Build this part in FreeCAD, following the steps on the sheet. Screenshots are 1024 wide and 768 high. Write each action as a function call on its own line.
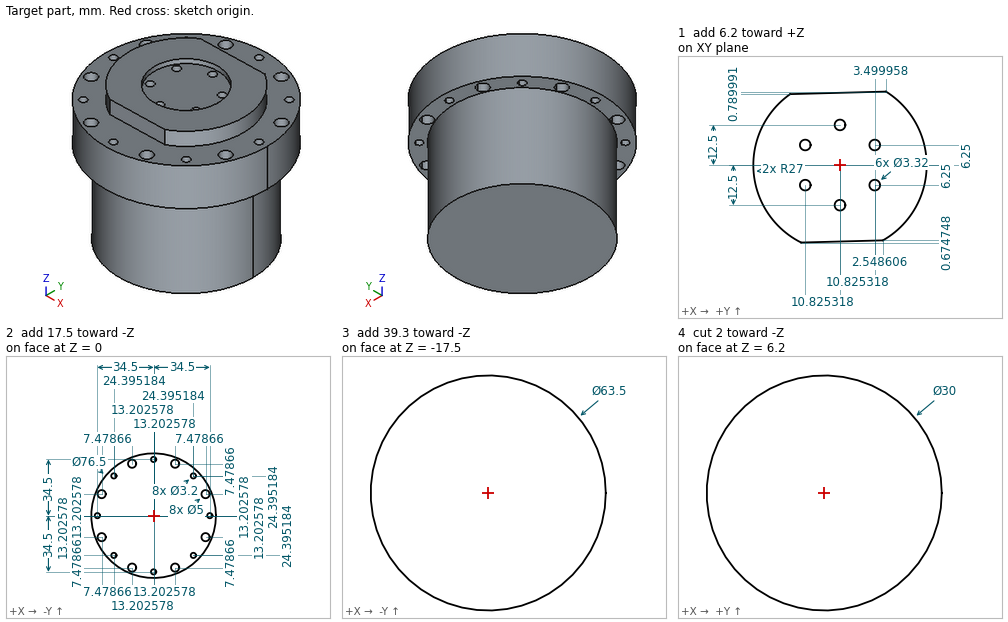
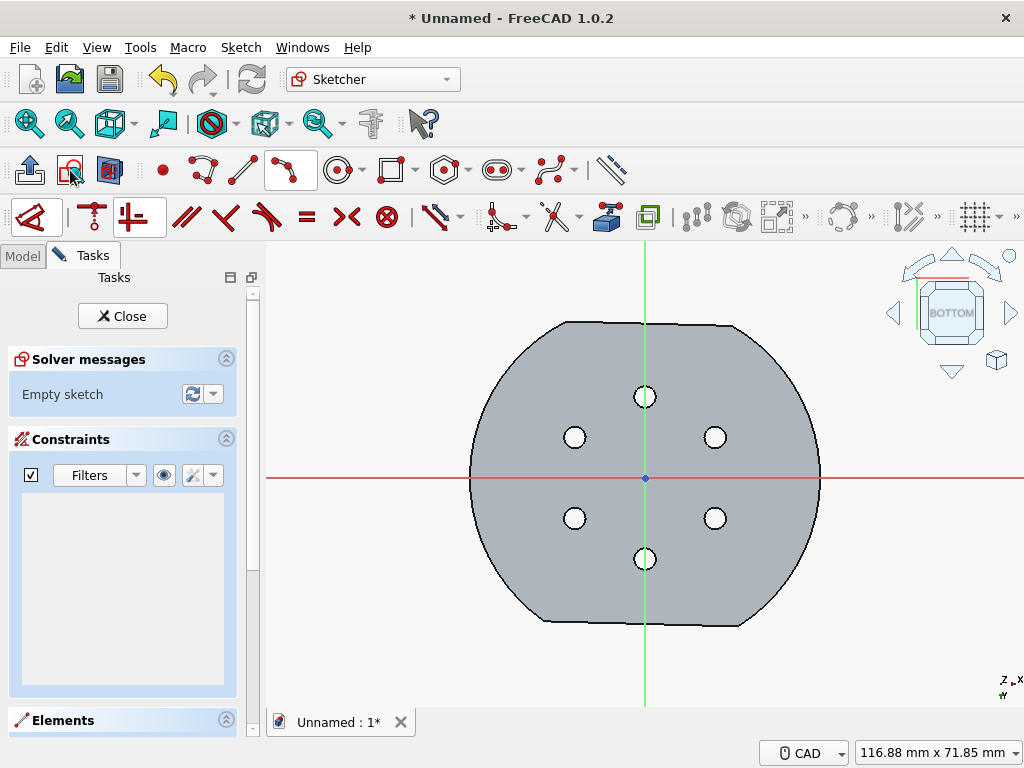
scroll(493, 469, down, 3)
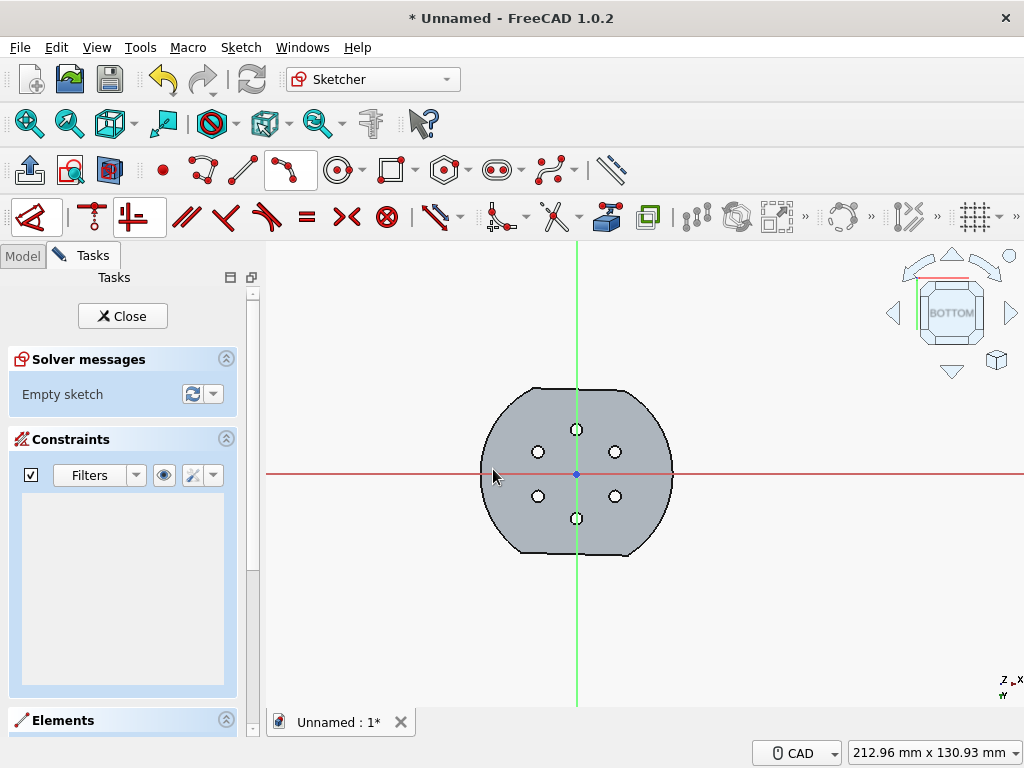
key(g)
key(c)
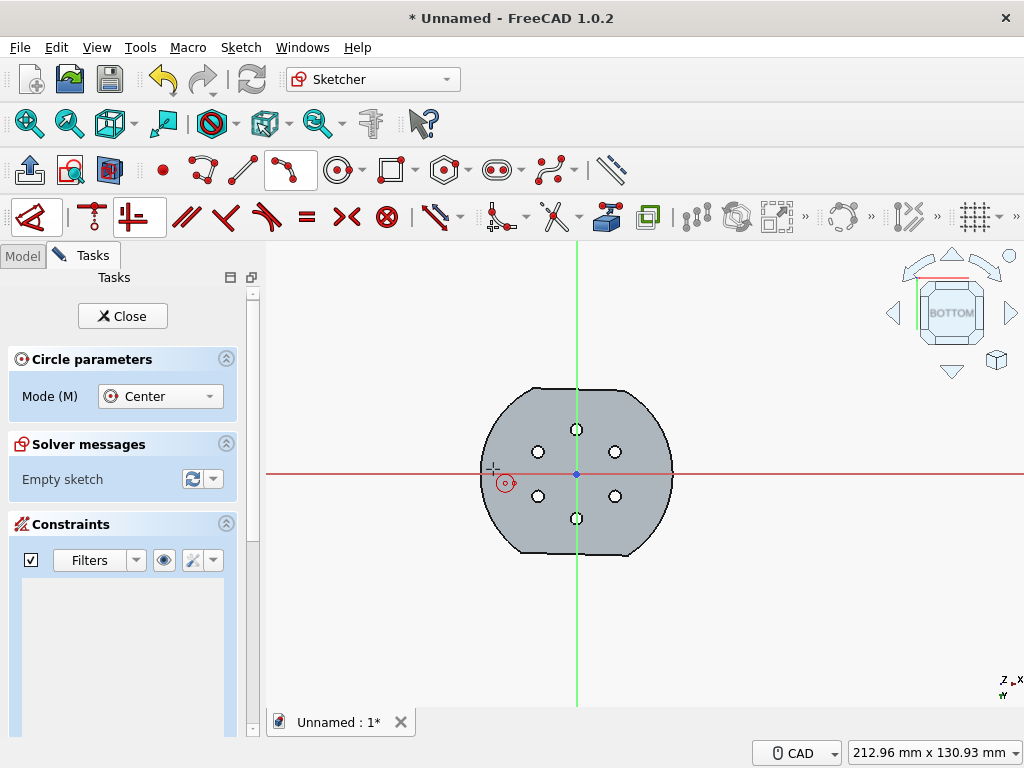
click(577, 474)
move(673, 378)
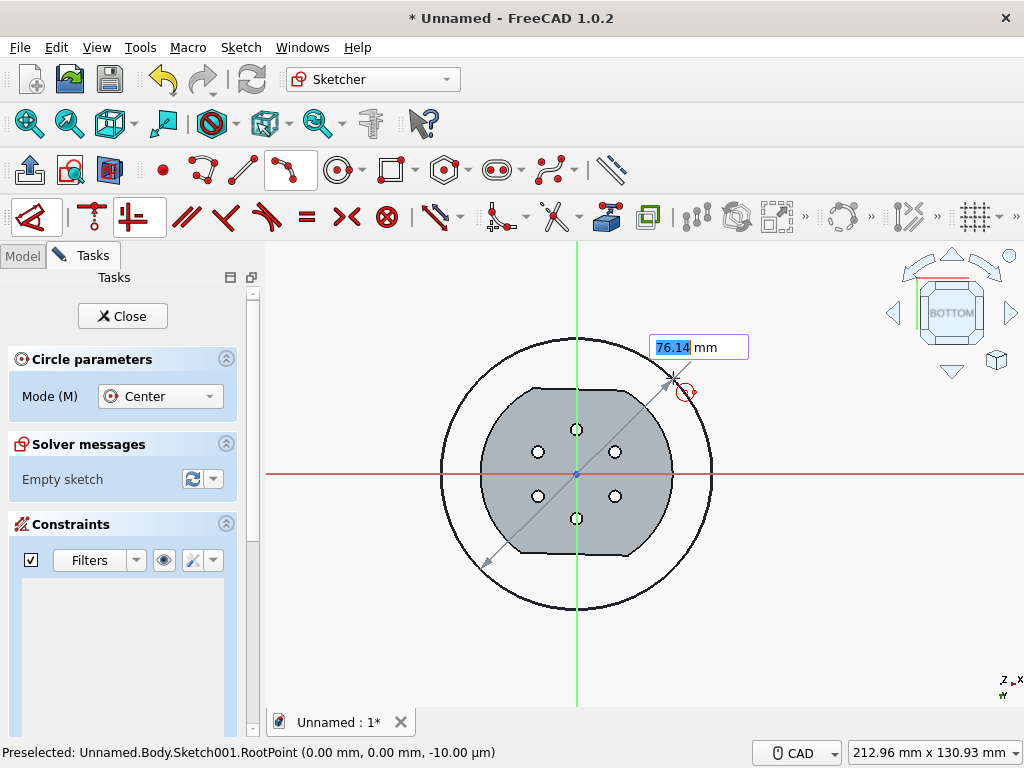
text(76.5)
key(Return)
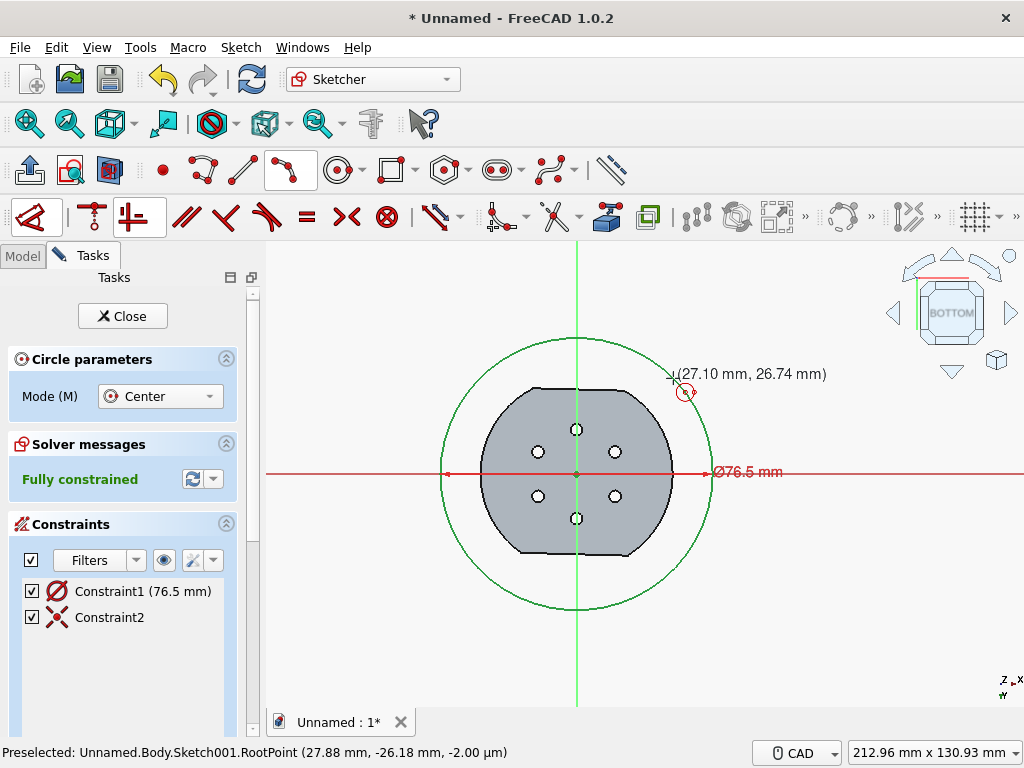
scroll(663, 387, up, 7)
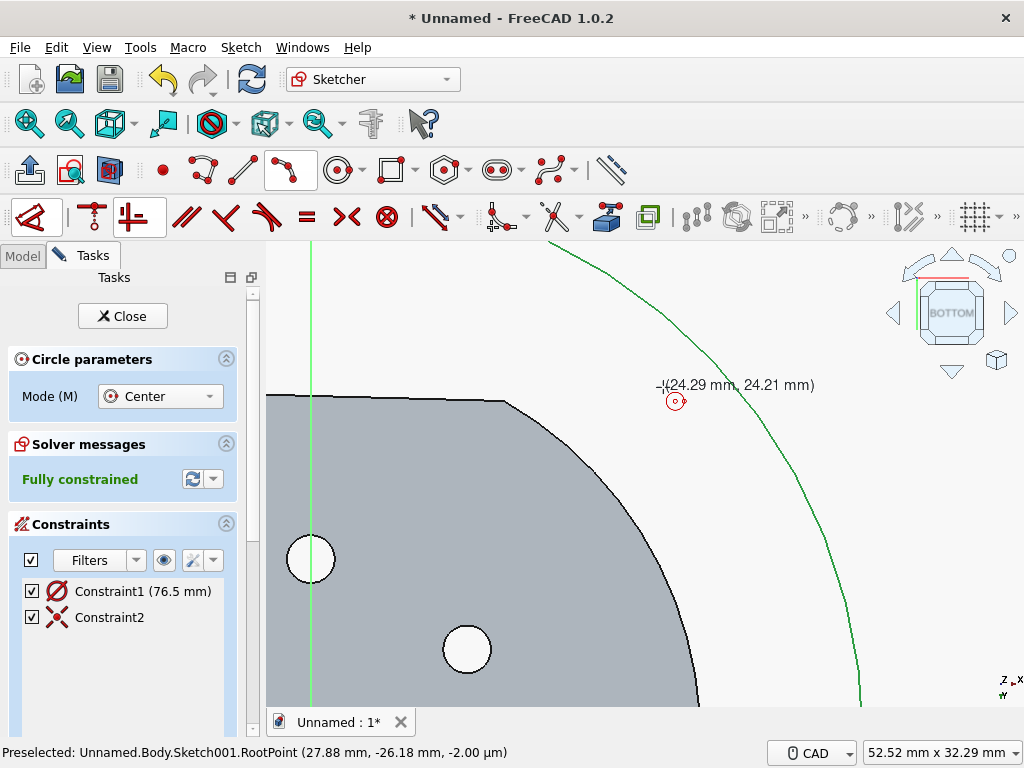
scroll(663, 387, down, 7)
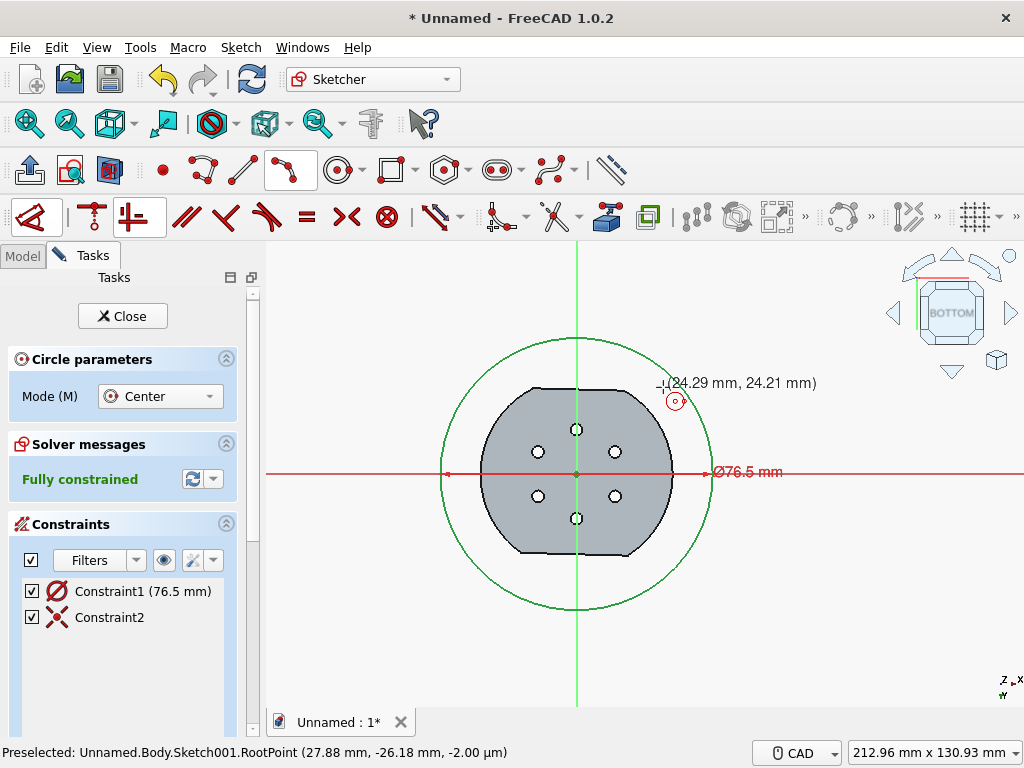
click(663, 387)
move(659, 391)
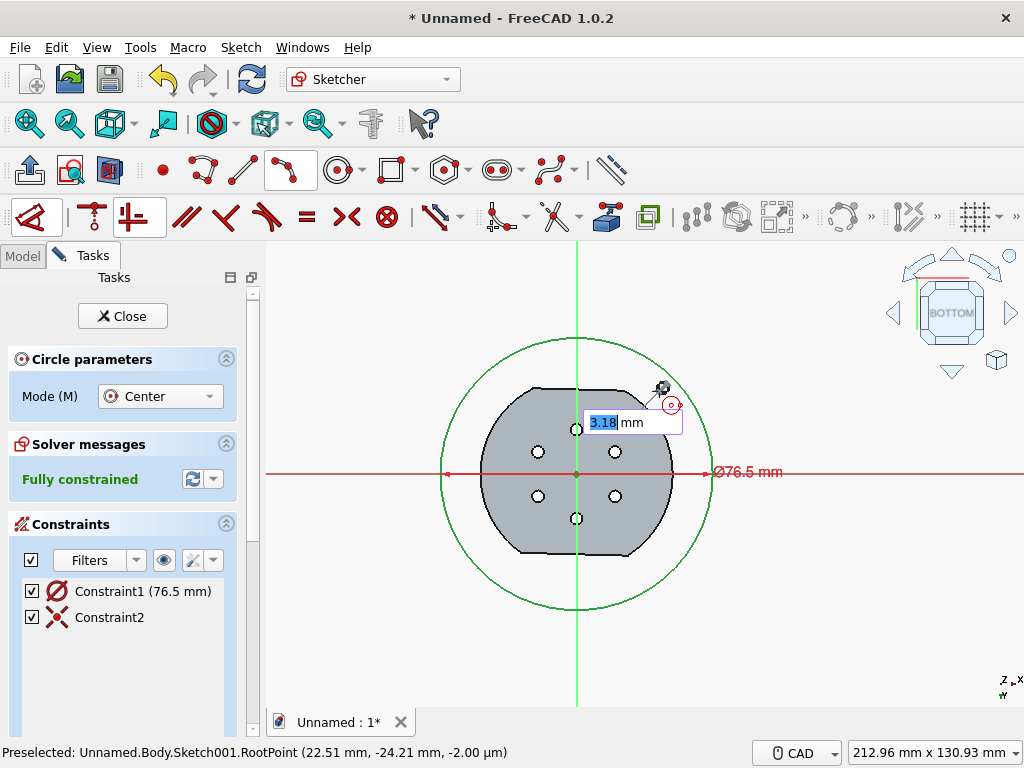
text(3.2)
key(Return)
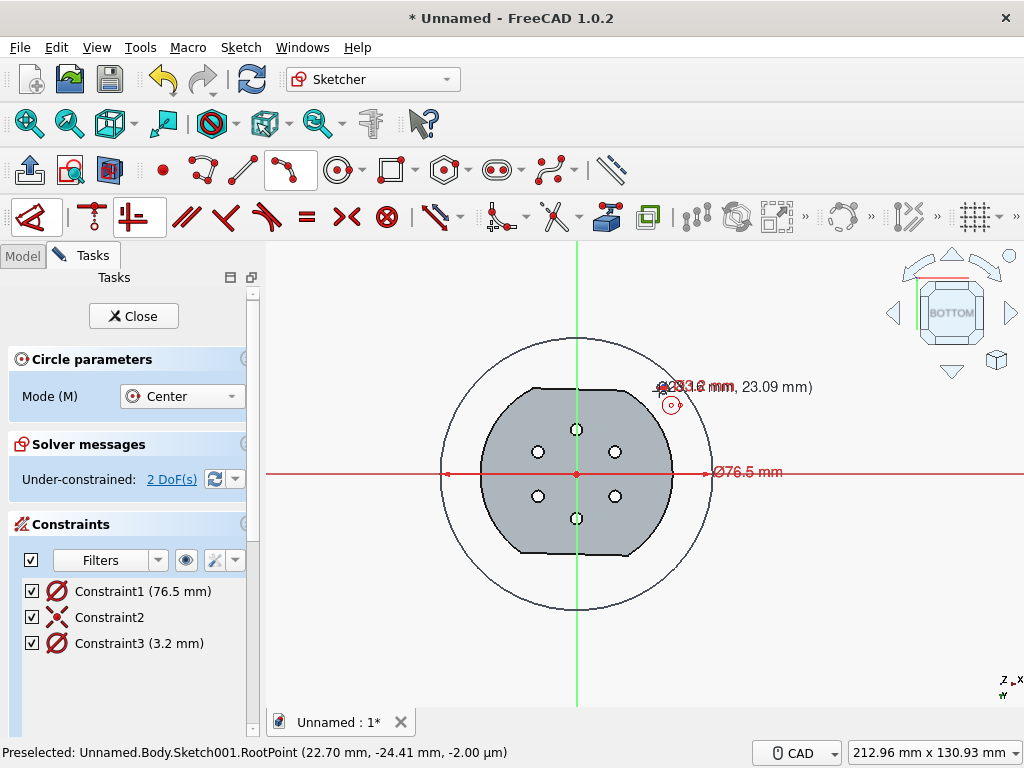
scroll(624, 361, up, 5)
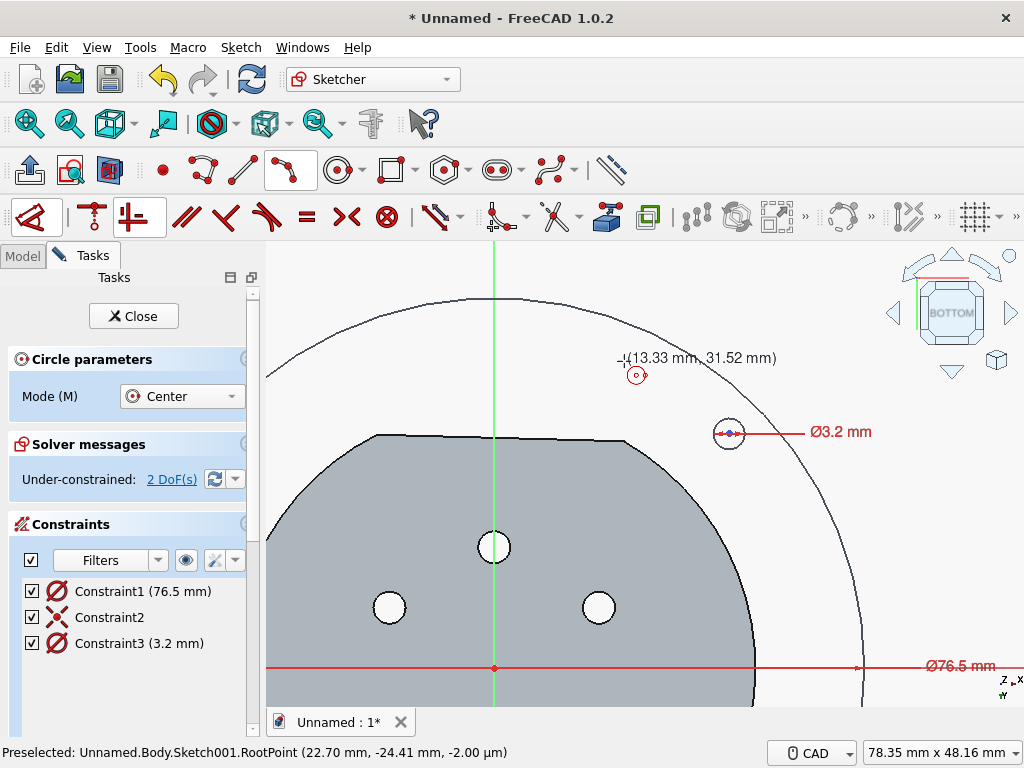
click(622, 360)
move(605, 343)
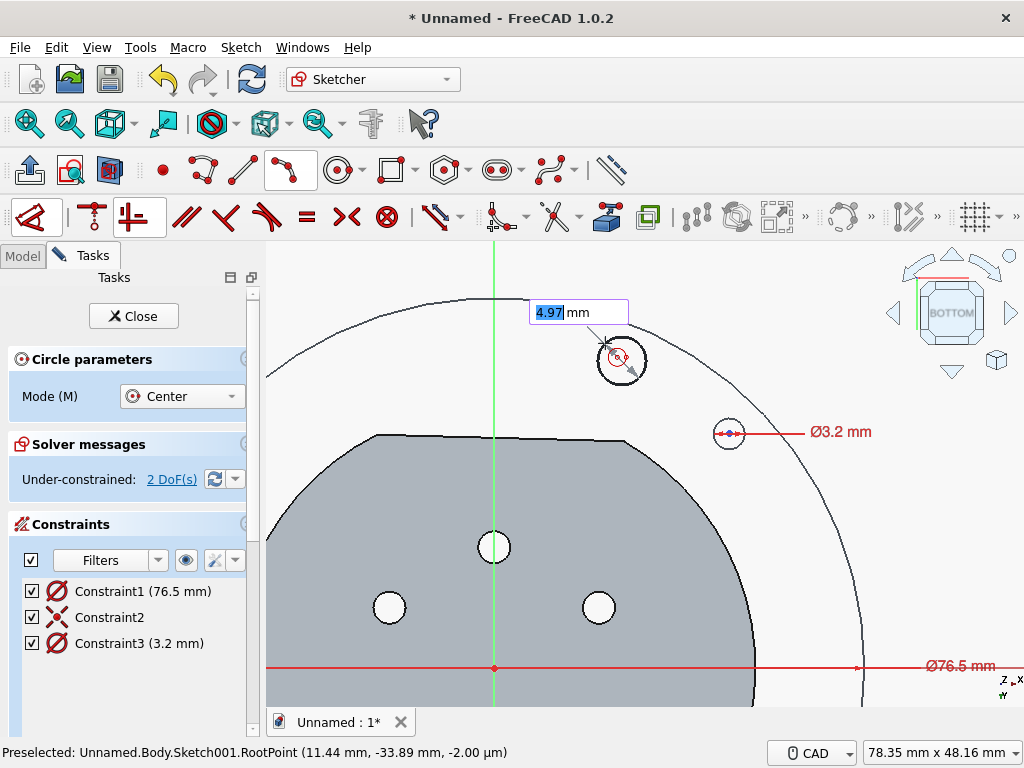
text(5)
key(Return)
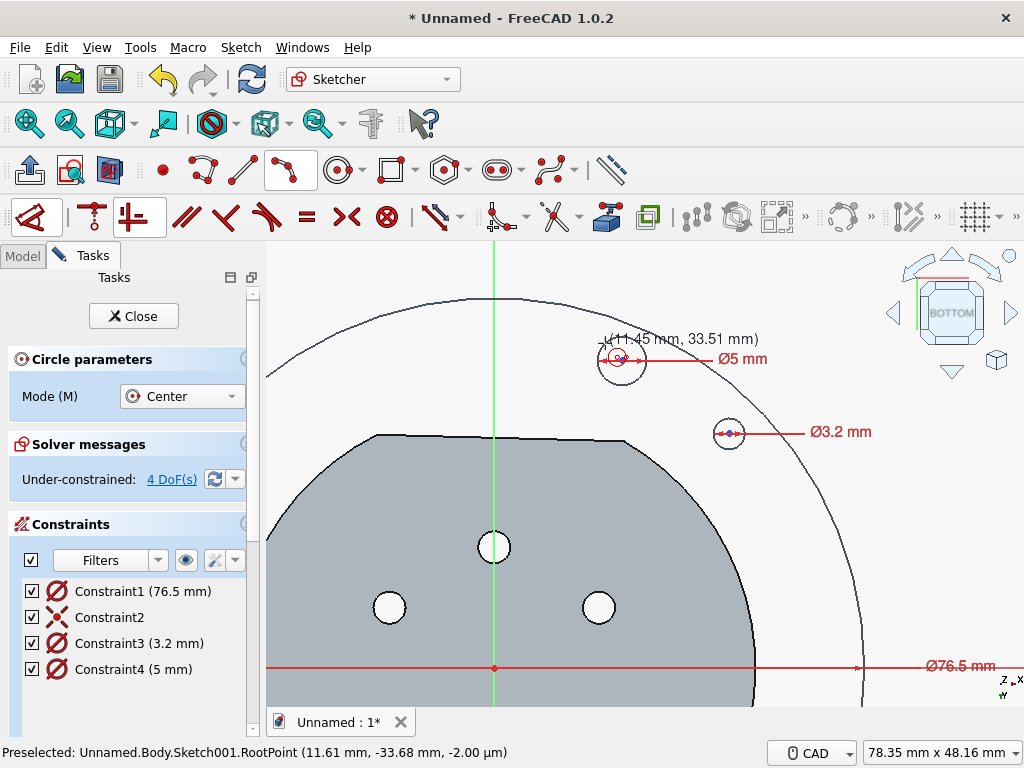
click(803, 540)
move(786, 523)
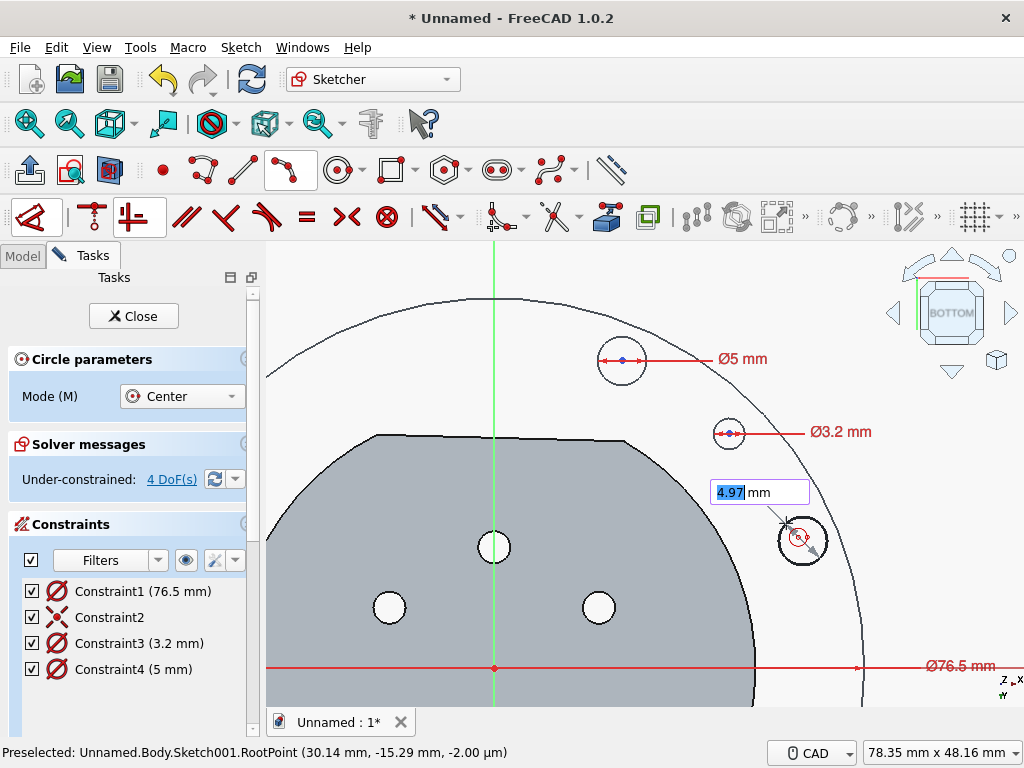
text(5)
key(Return)